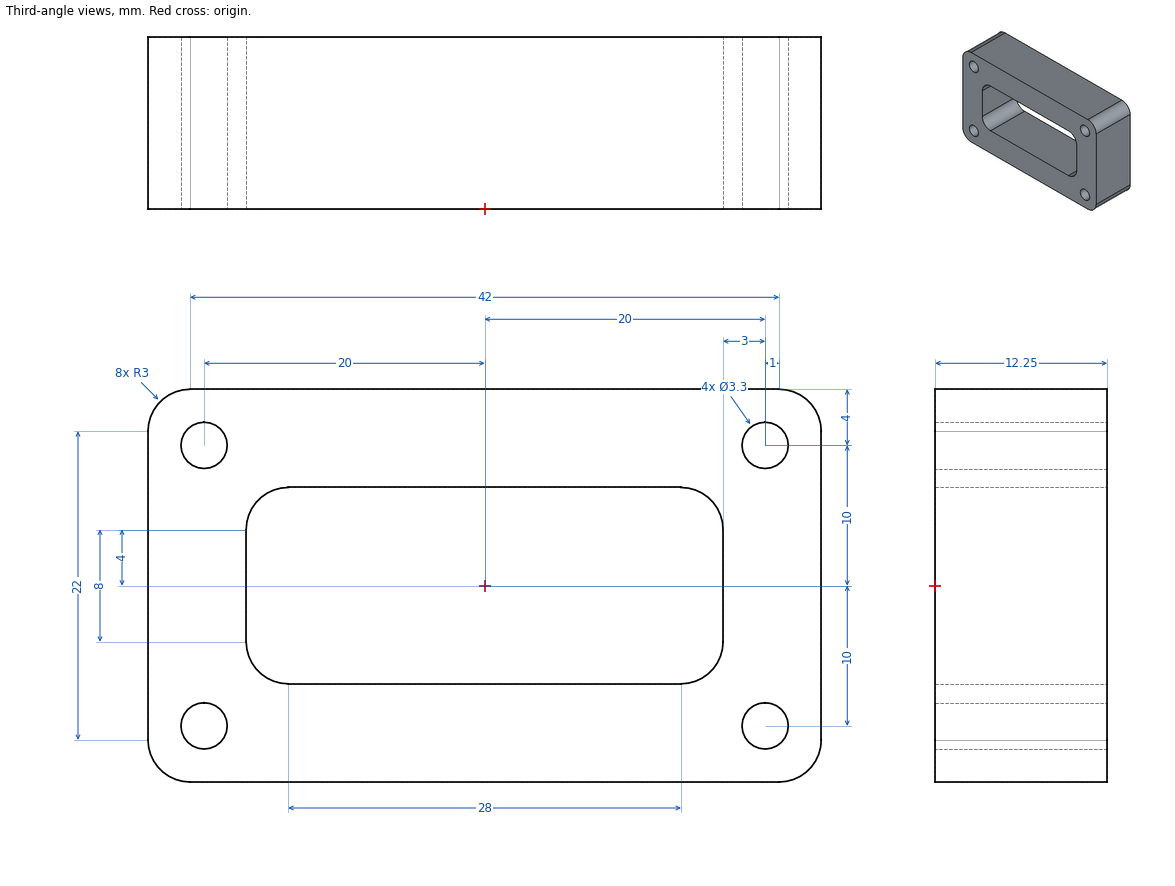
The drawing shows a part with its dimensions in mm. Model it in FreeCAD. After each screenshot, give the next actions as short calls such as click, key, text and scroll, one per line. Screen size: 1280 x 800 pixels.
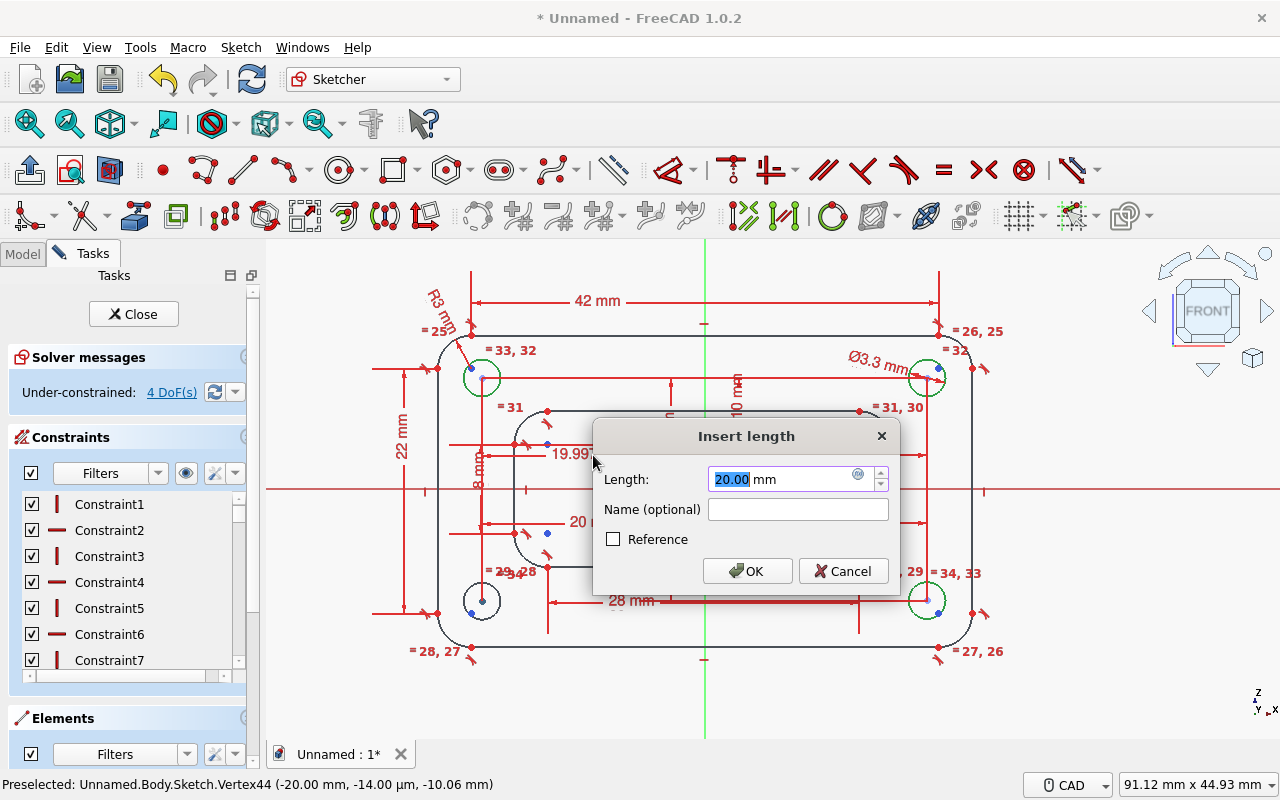
text(20)
key(Return)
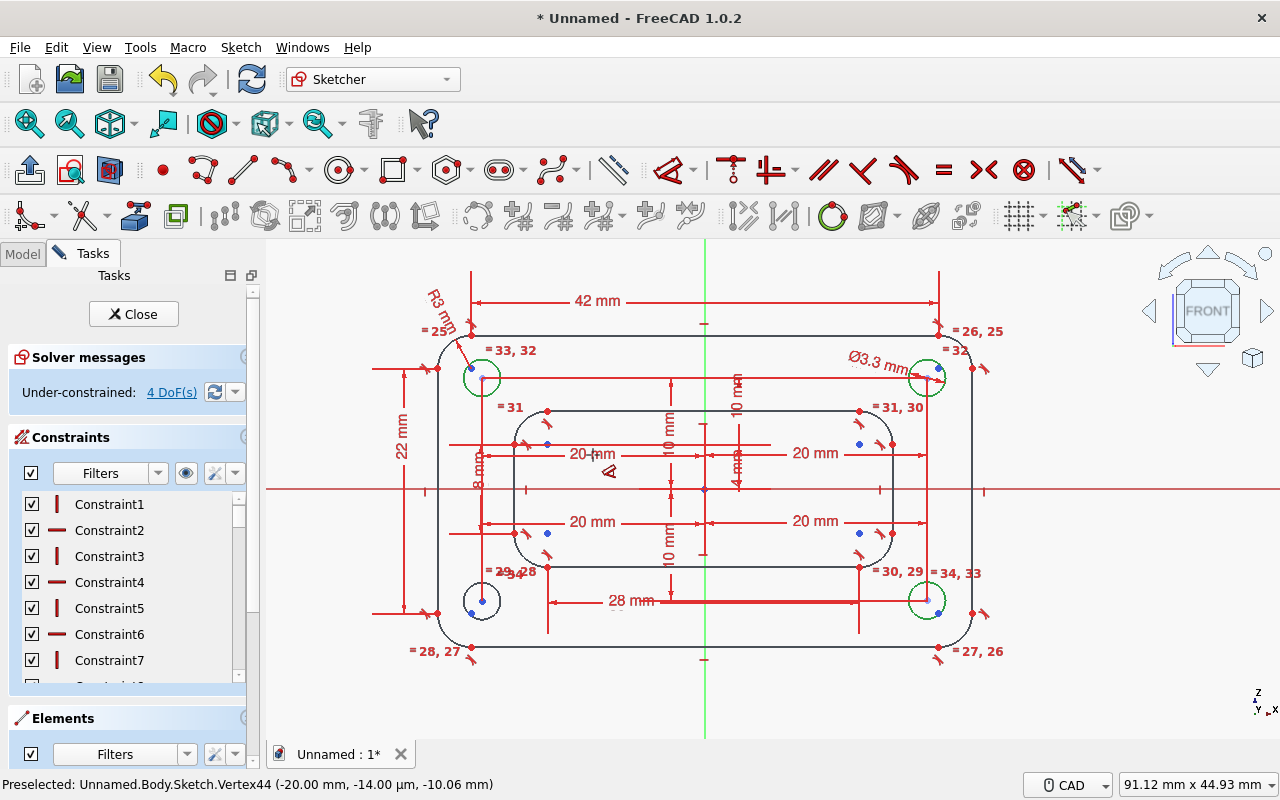
click(482, 601)
click(739, 520)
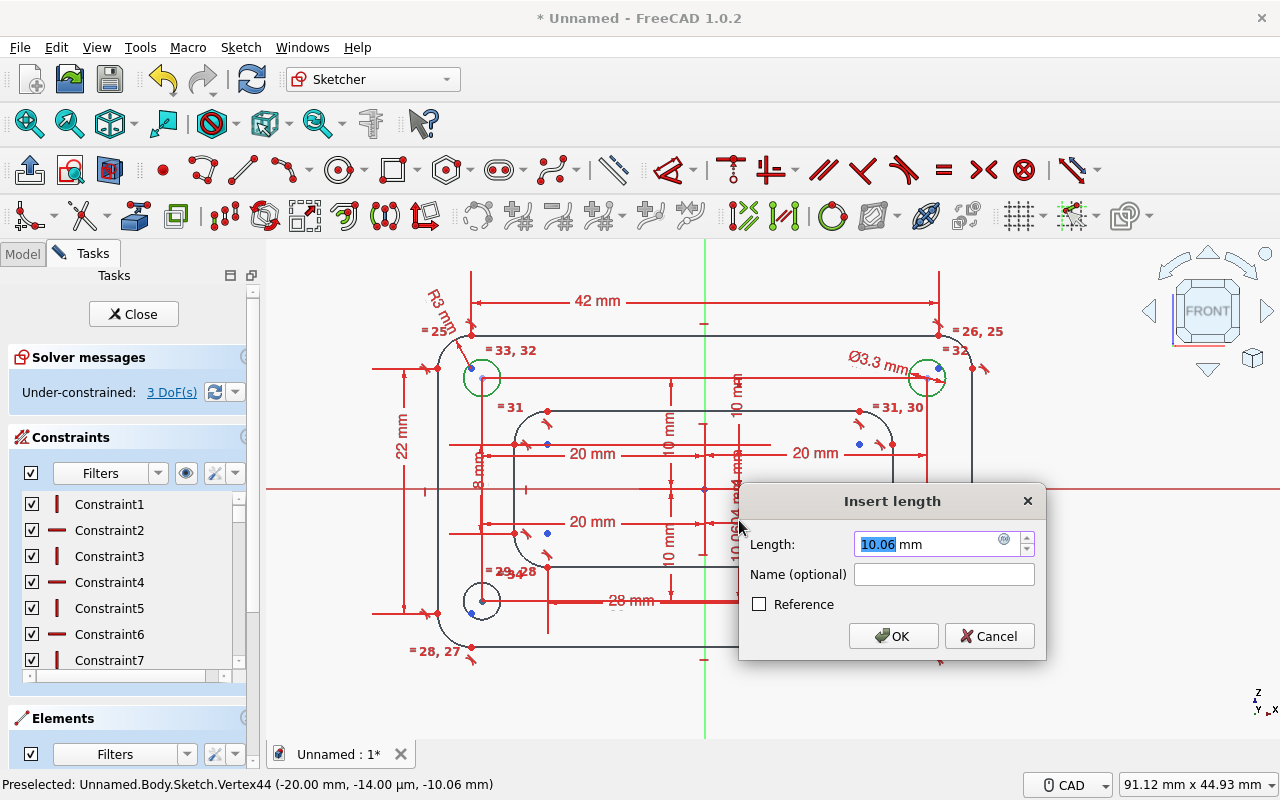
text(10)
key(Return)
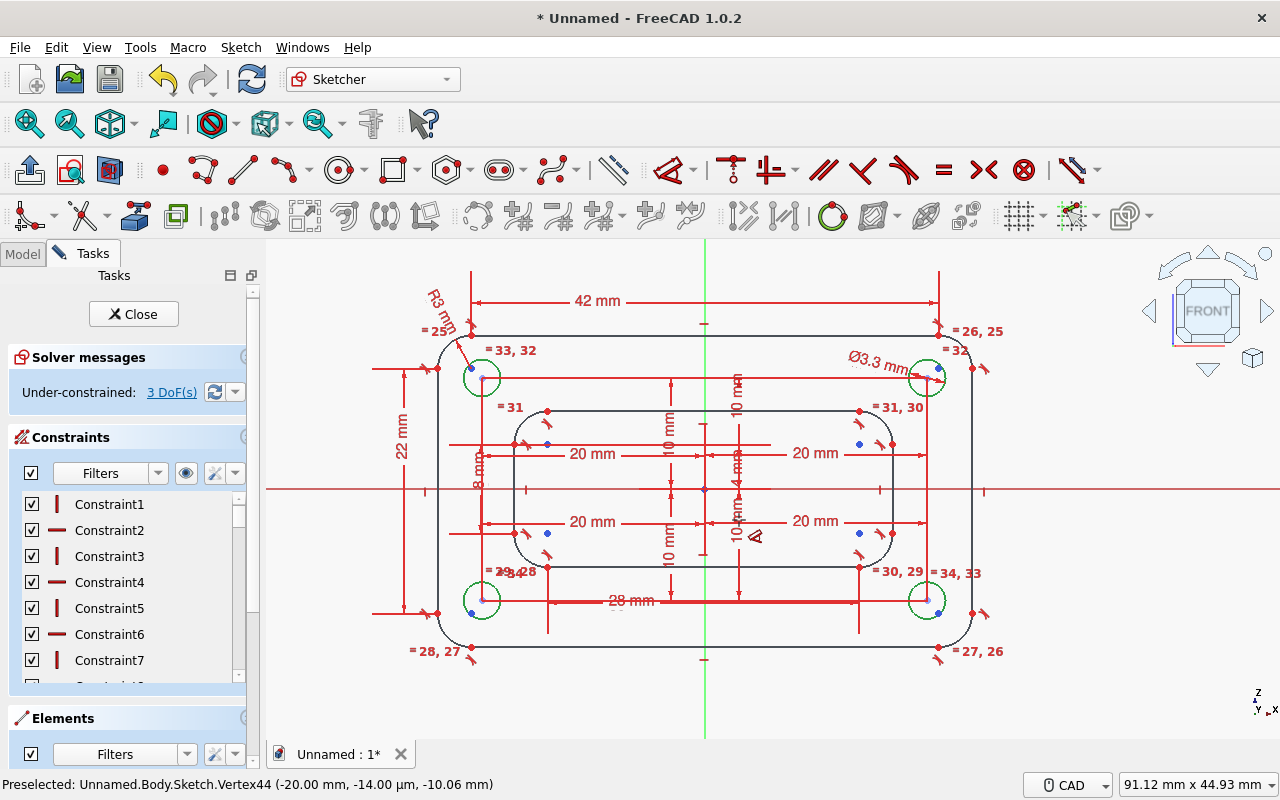
scroll(939, 336, up, 7)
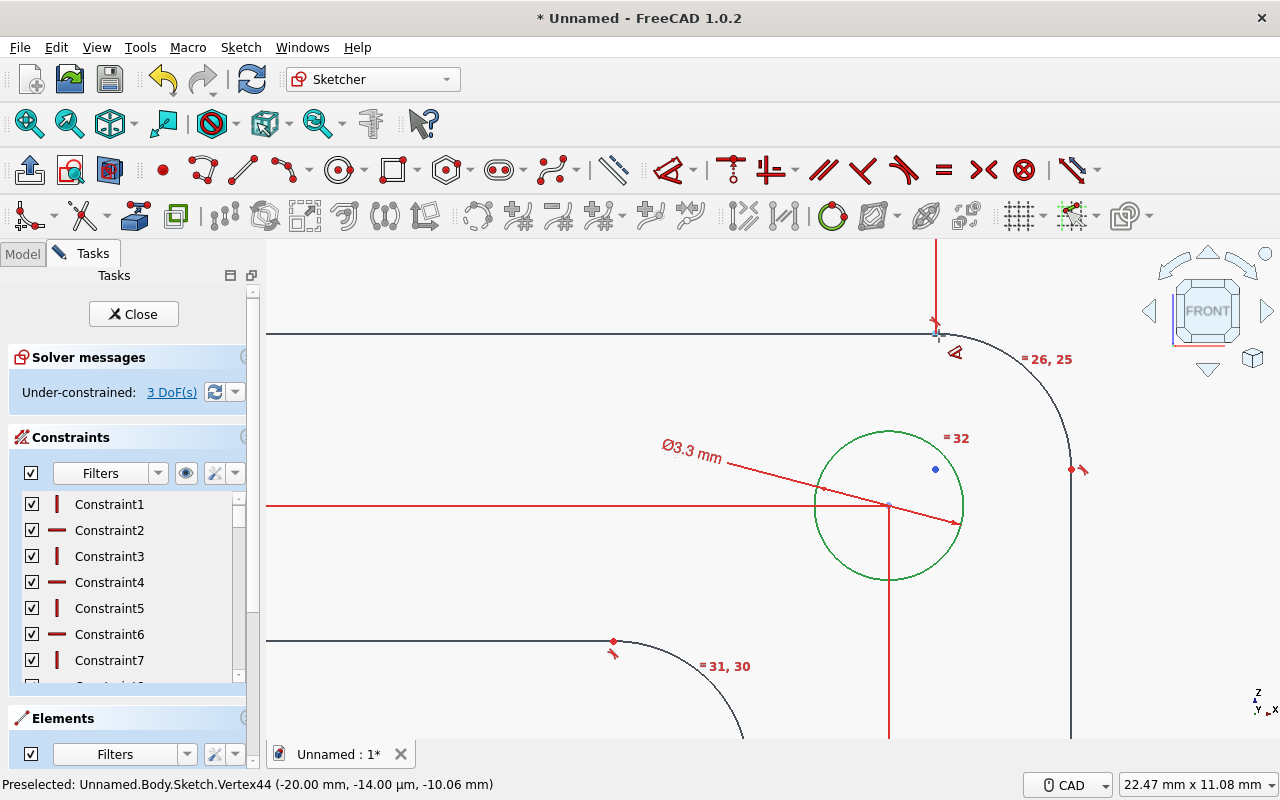
click(936, 334)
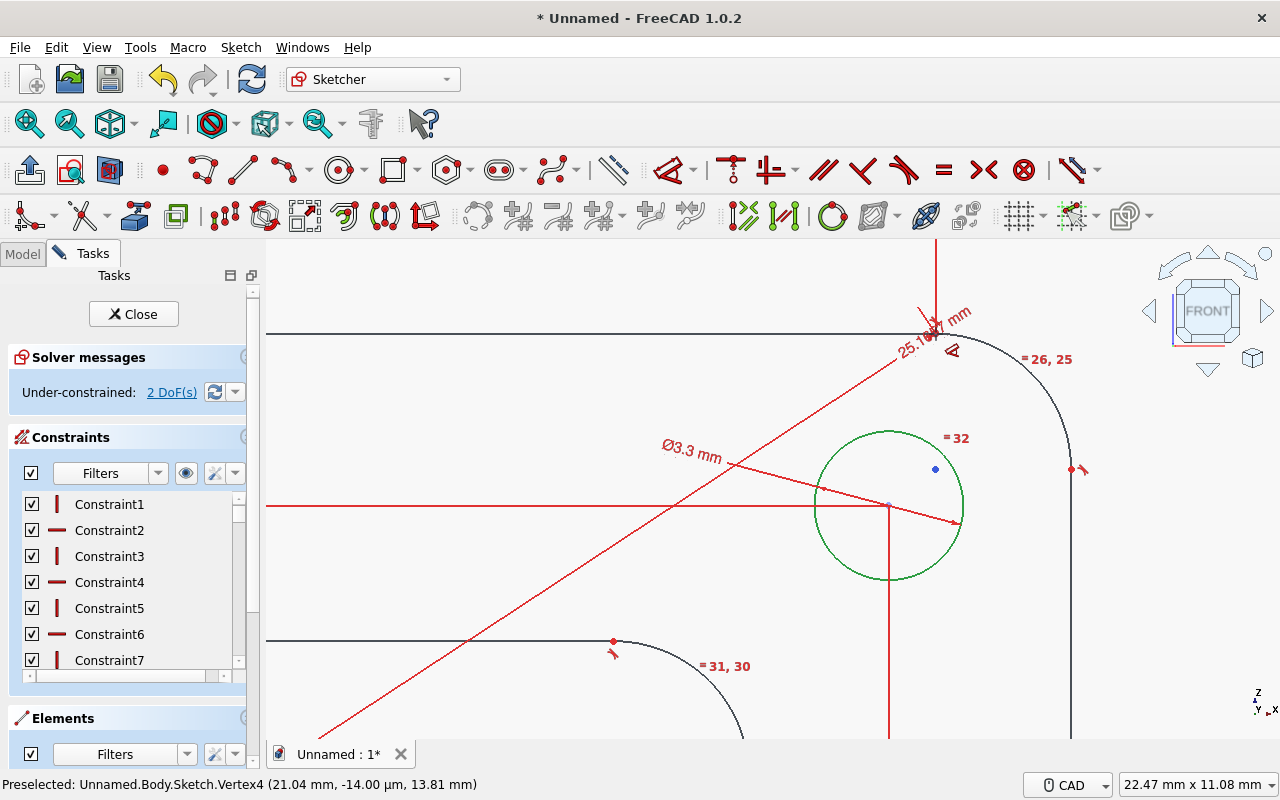
click(889, 506)
click(912, 300)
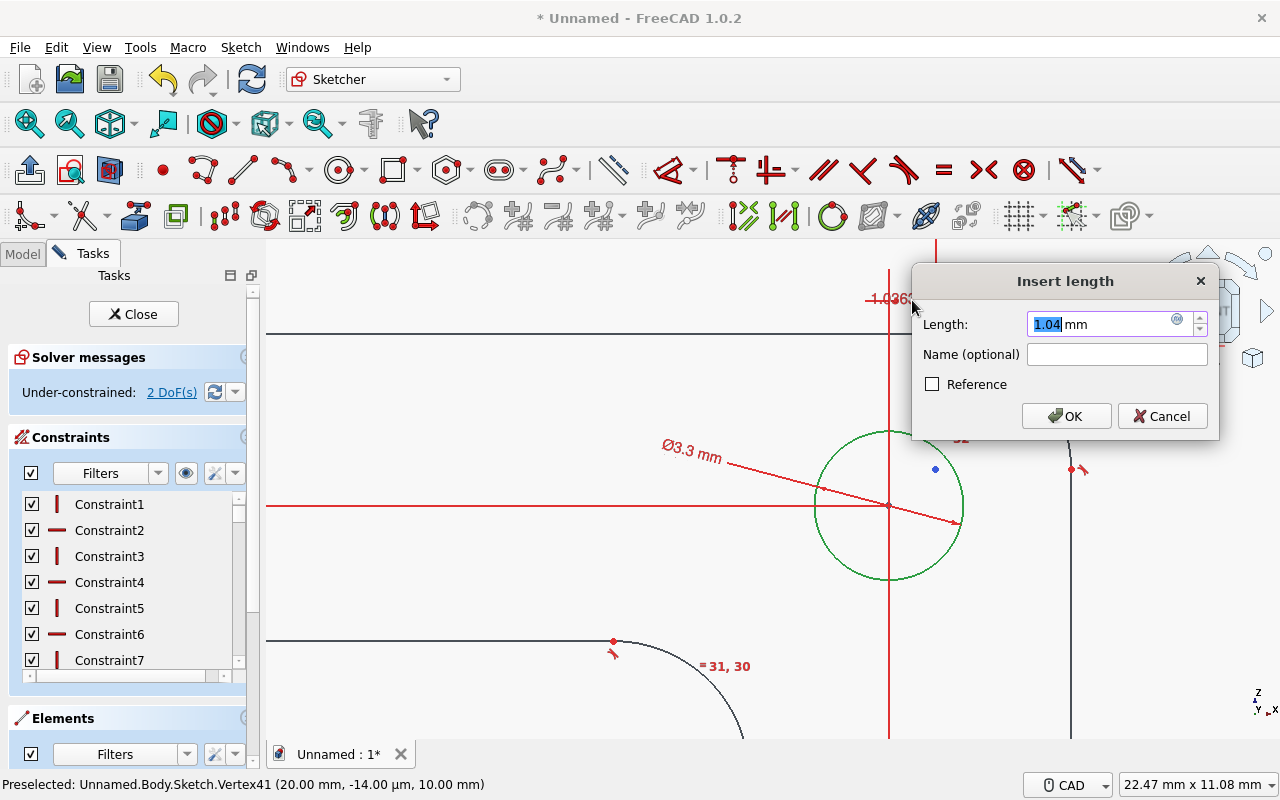
text(1)
key(Return)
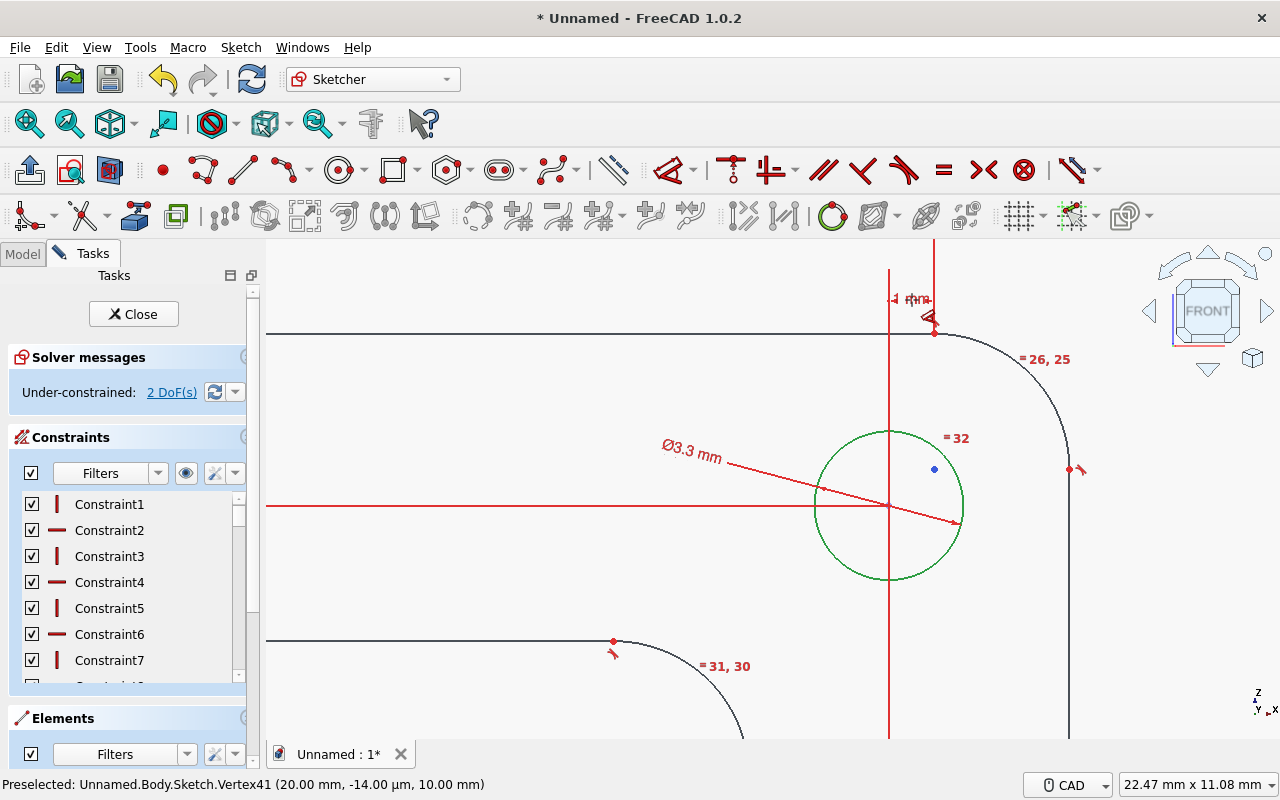
scroll(940, 336, down, 7)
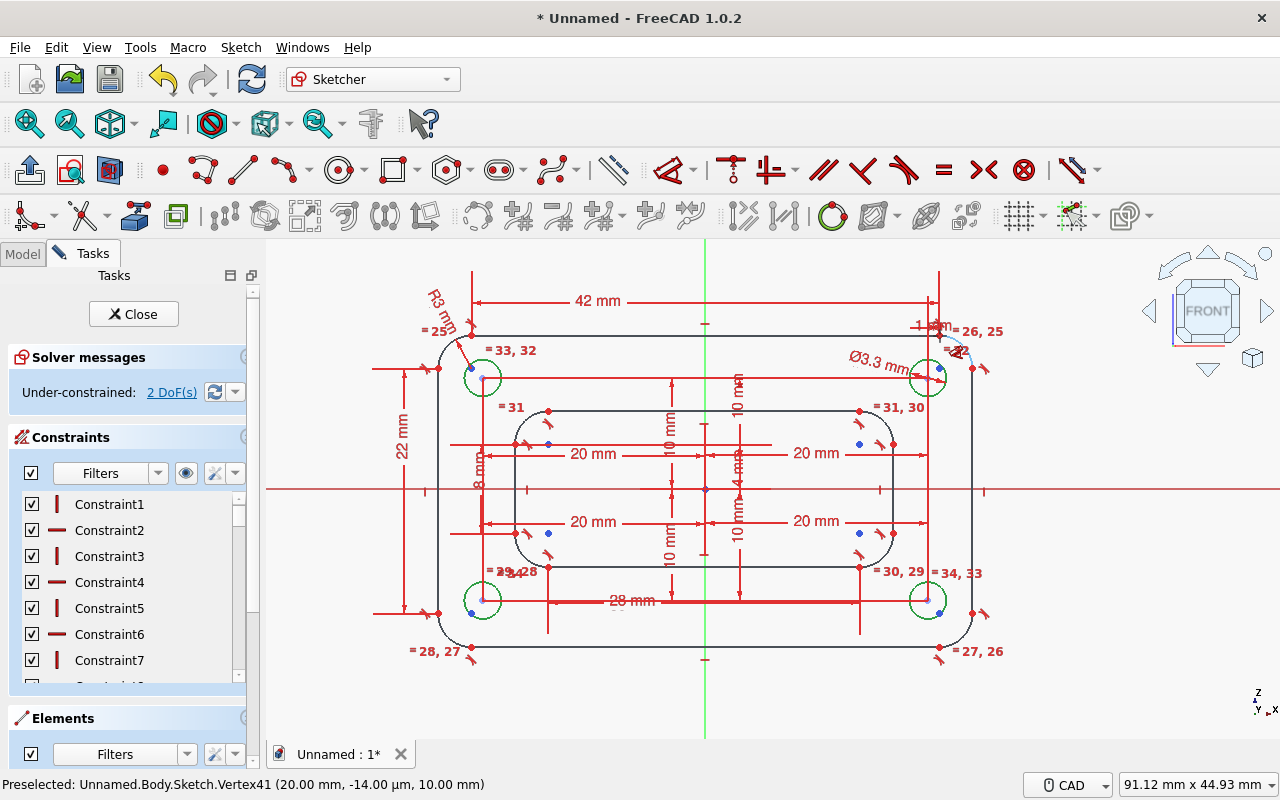
click(893, 445)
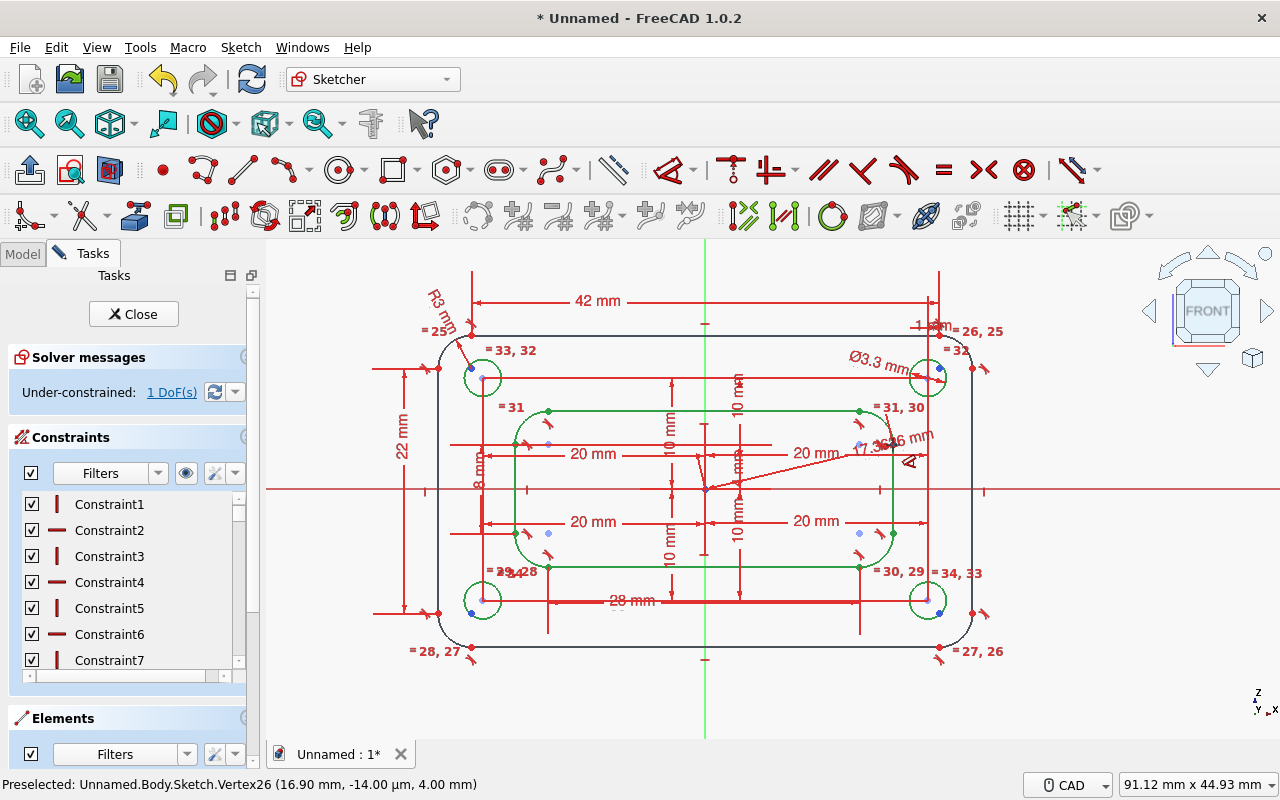
click(928, 378)
click(911, 503)